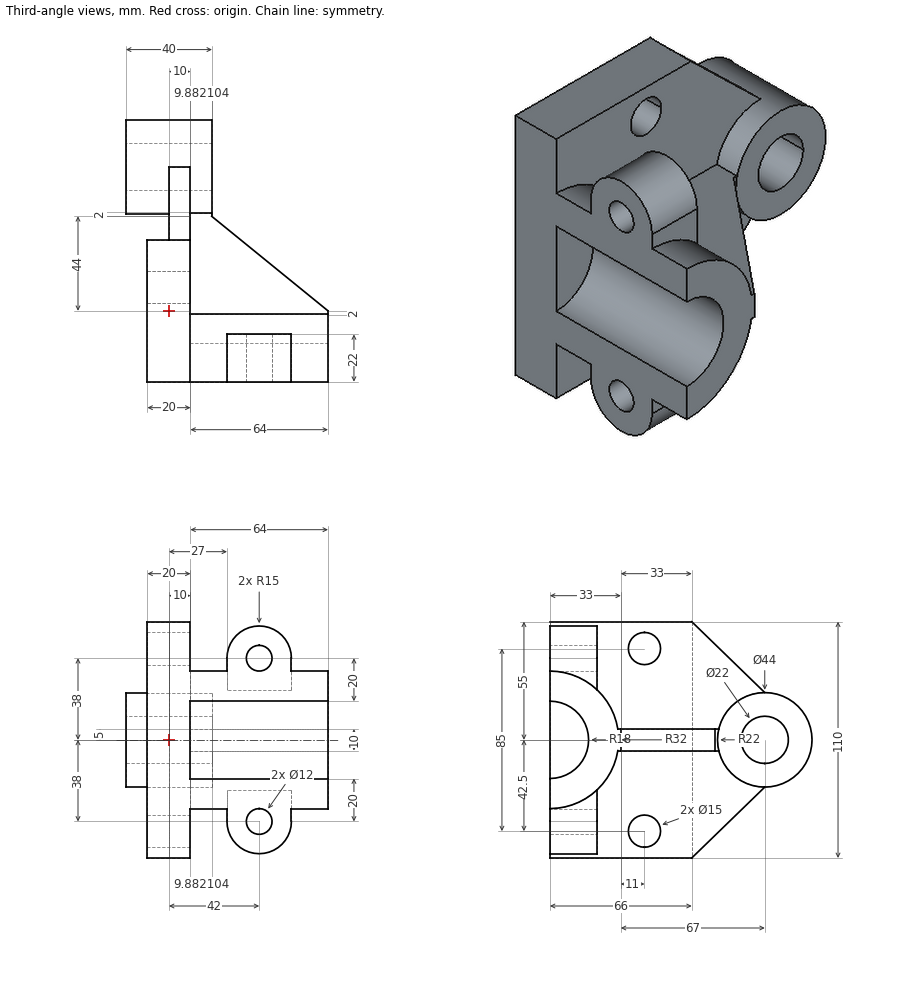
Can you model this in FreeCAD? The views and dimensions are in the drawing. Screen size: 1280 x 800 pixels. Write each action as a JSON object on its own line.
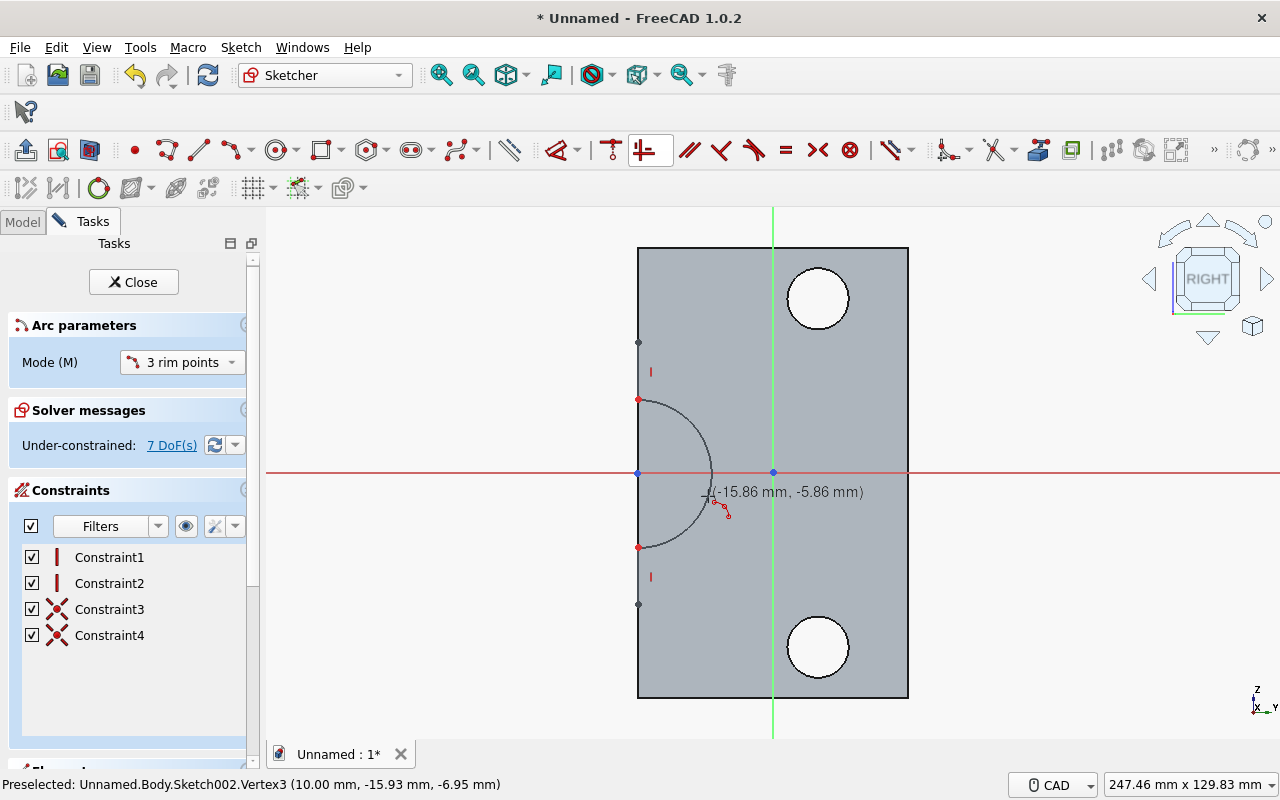
{"action": "left_click", "coordinate": [638, 605]}
{"action": "left_click", "coordinate": [638, 343]}
{"action": "left_click", "coordinate": [744, 550]}
{"action": "key", "text": "Escape"}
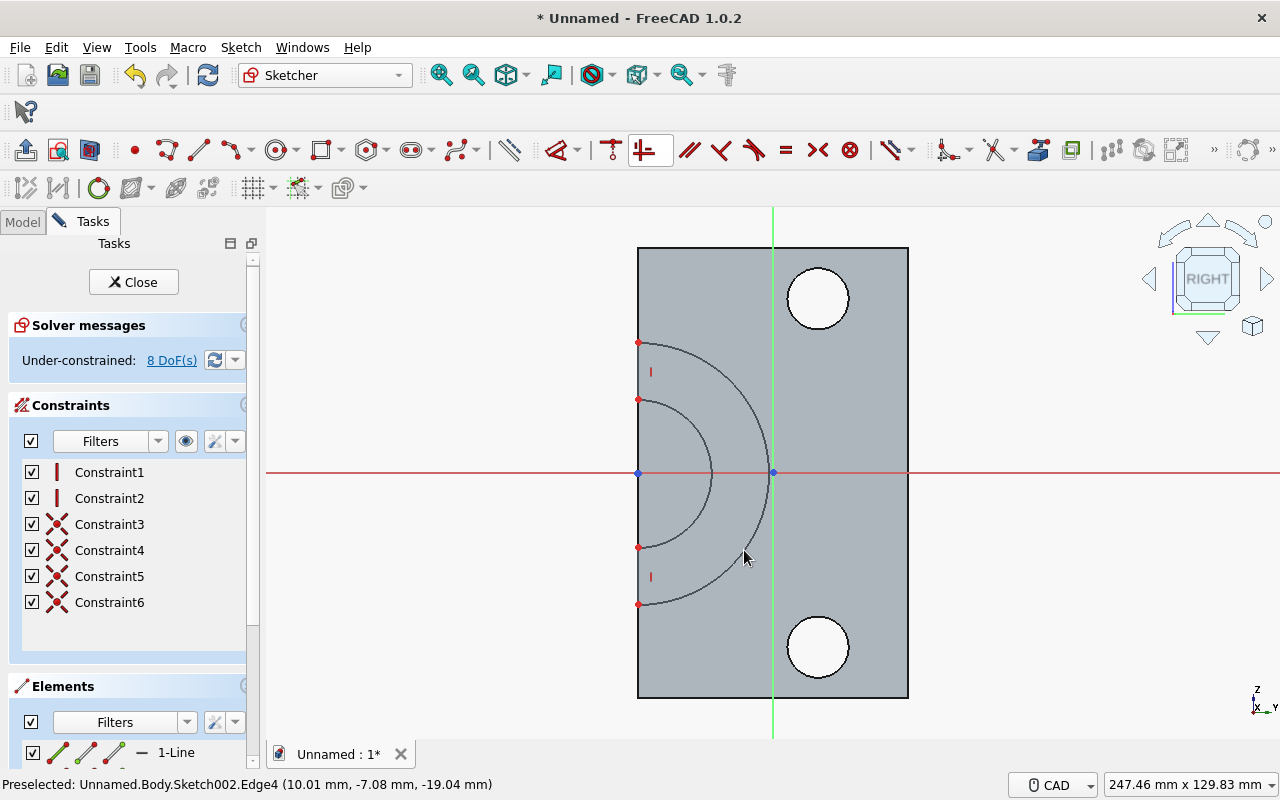
{"action": "left_click", "coordinate": [698, 517]}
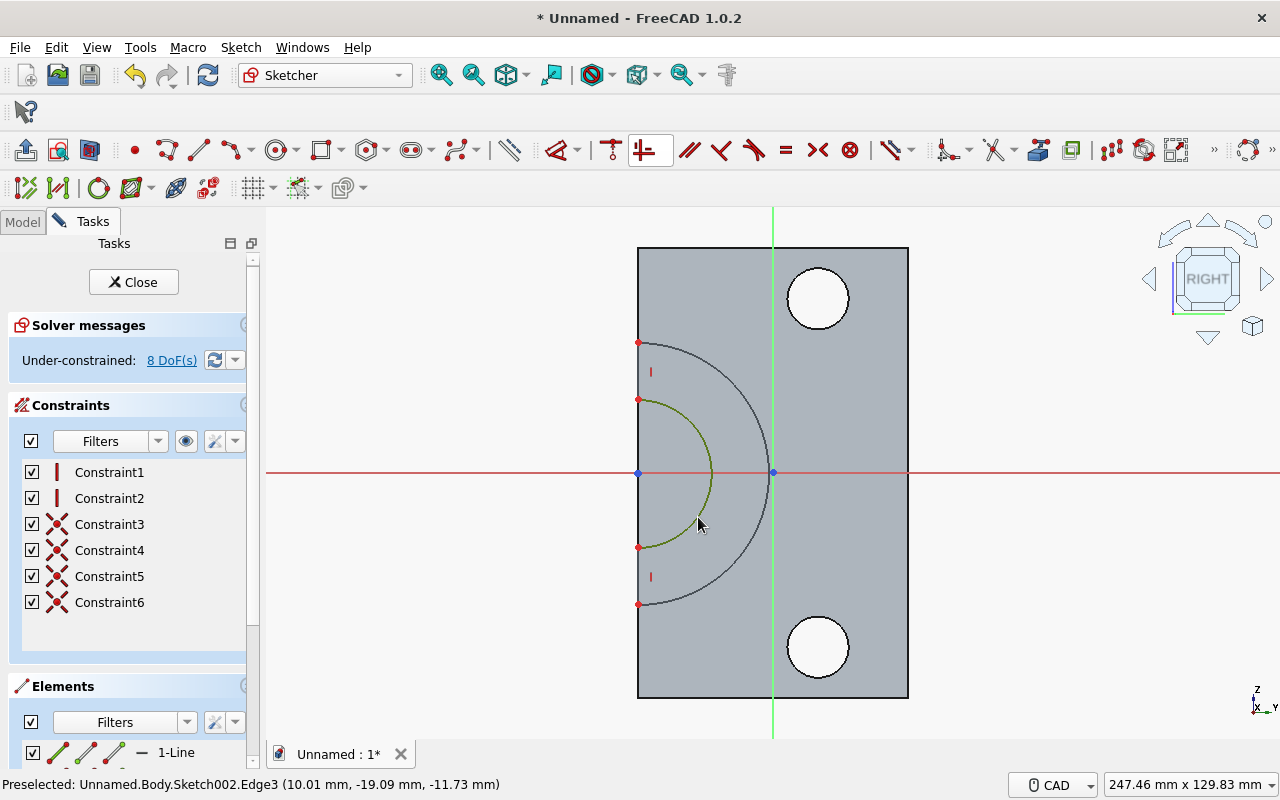
{"action": "left_click", "coordinate": [744, 551]}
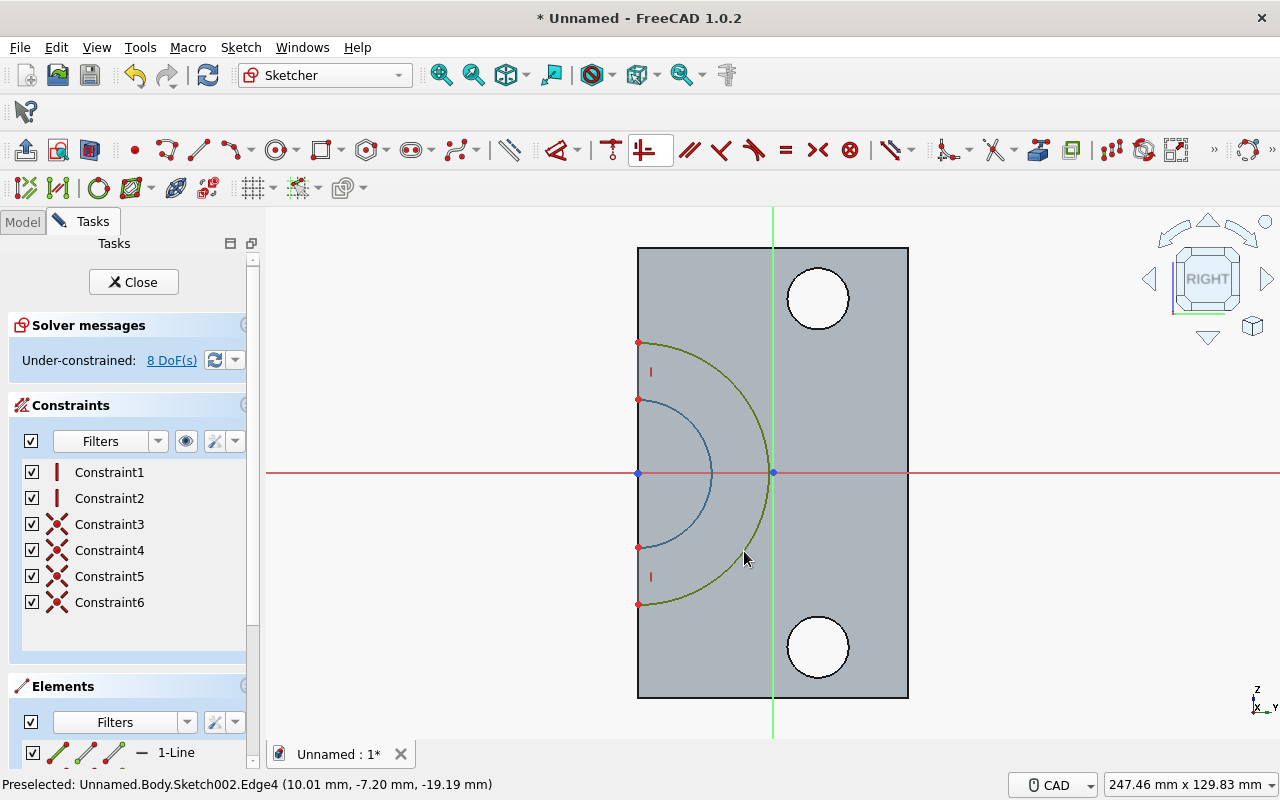
{"action": "left_click", "coordinate": [612, 150]}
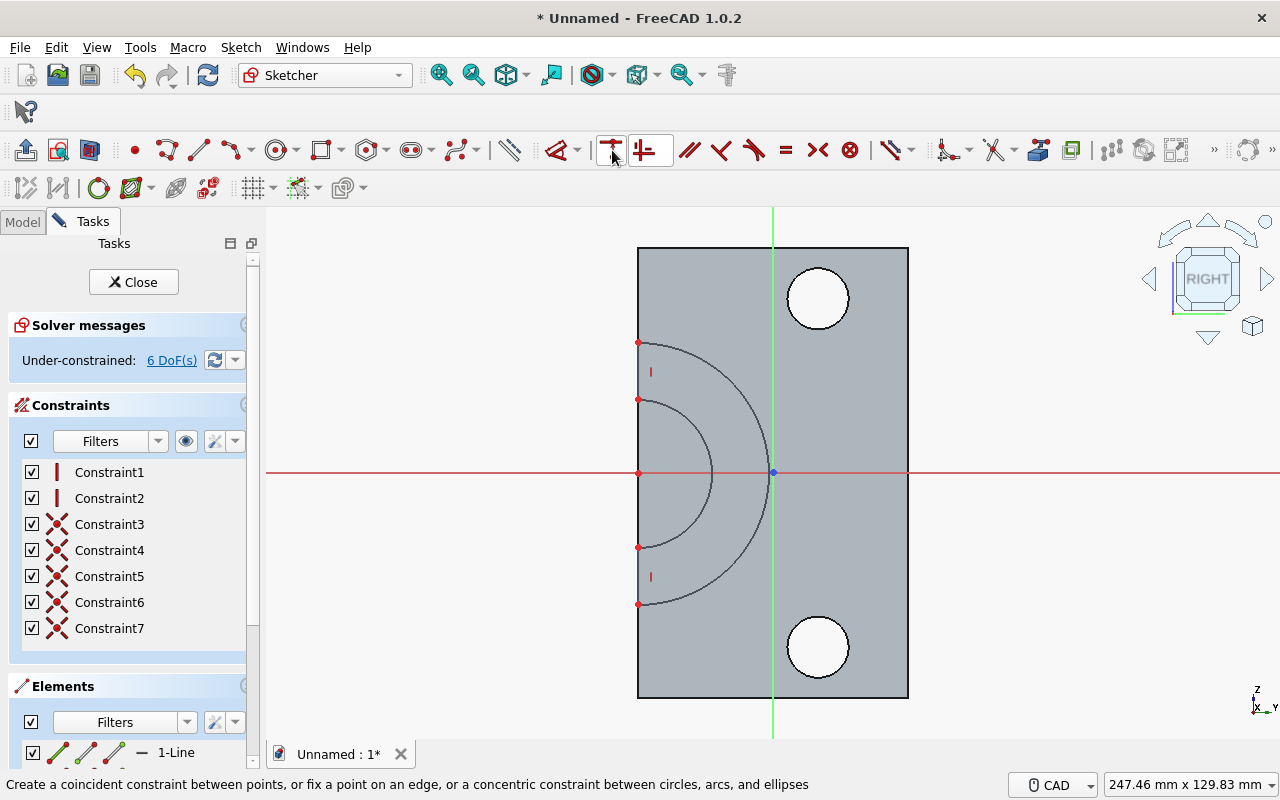
{"action": "left_click", "coordinate": [638, 474]}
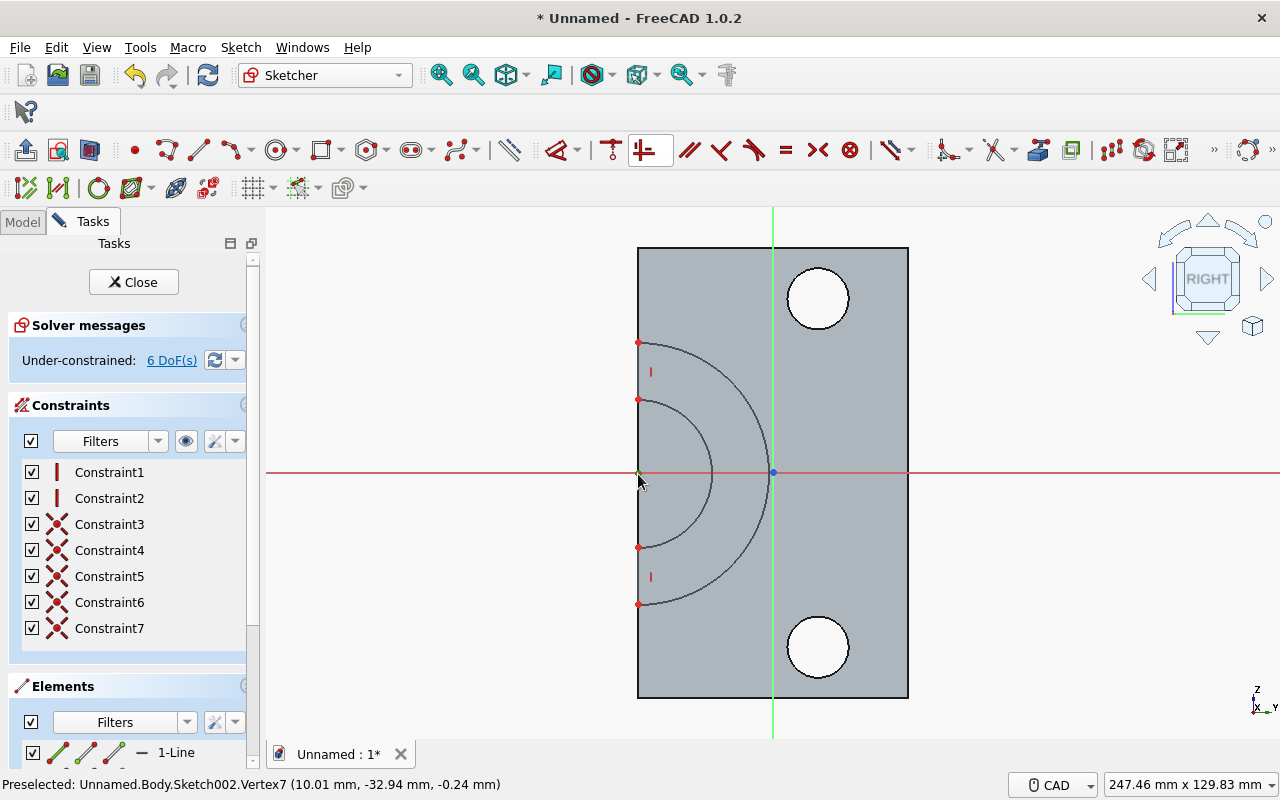
{"action": "left_click", "coordinate": [353, 473]}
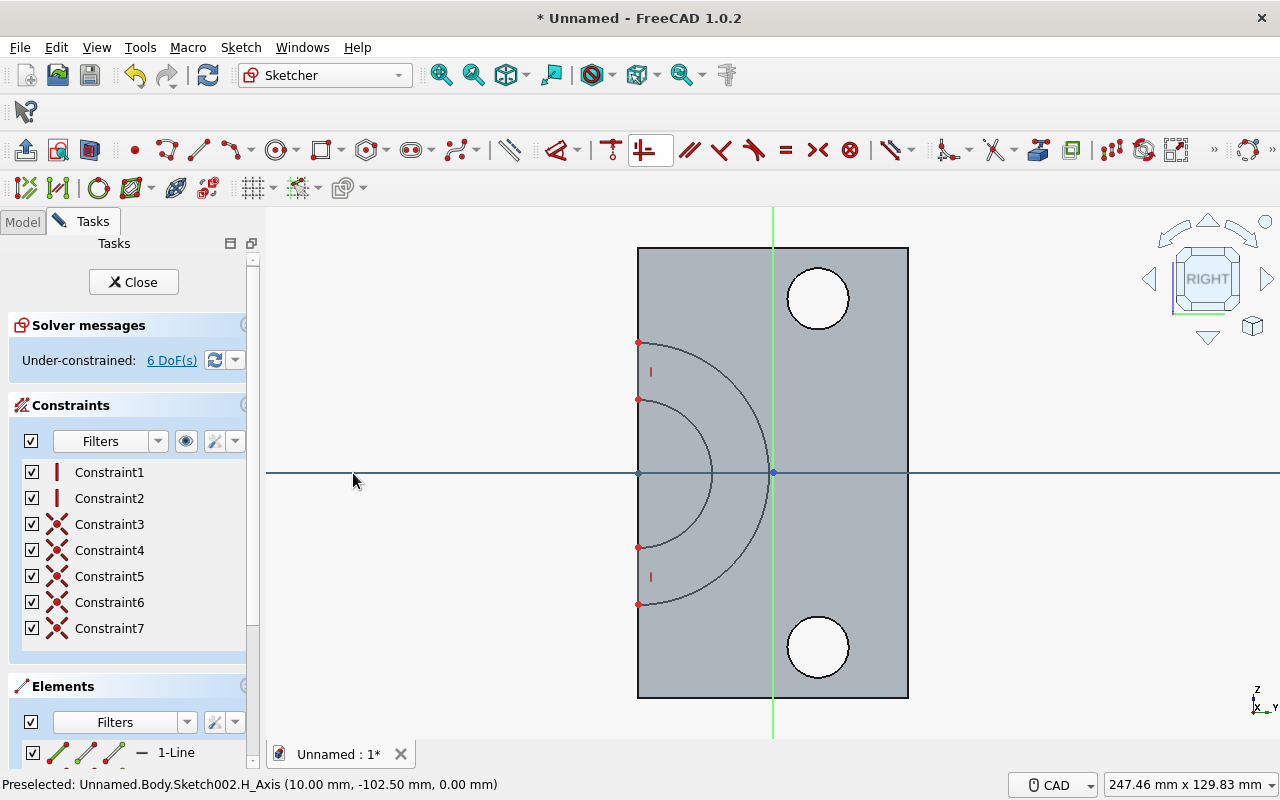
{"action": "key", "text": "c"}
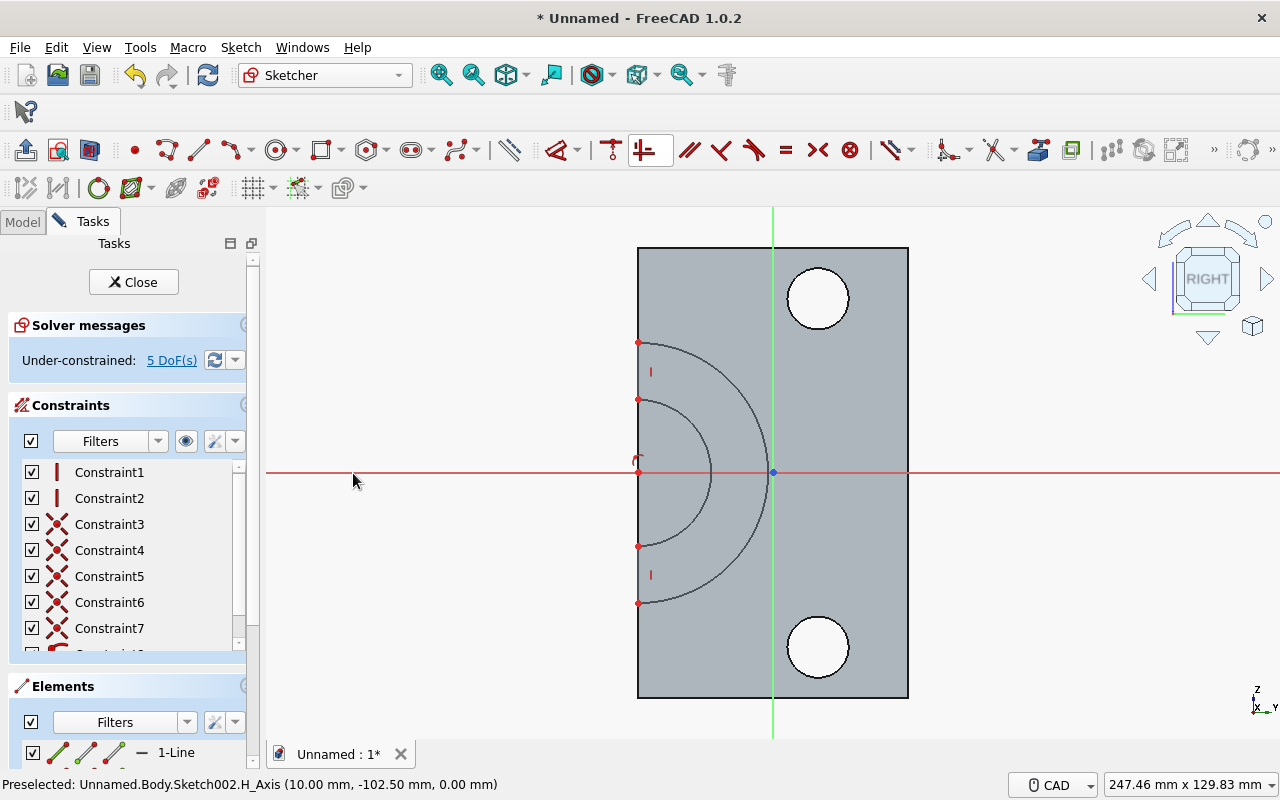
{"action": "left_click", "coordinate": [556, 150]}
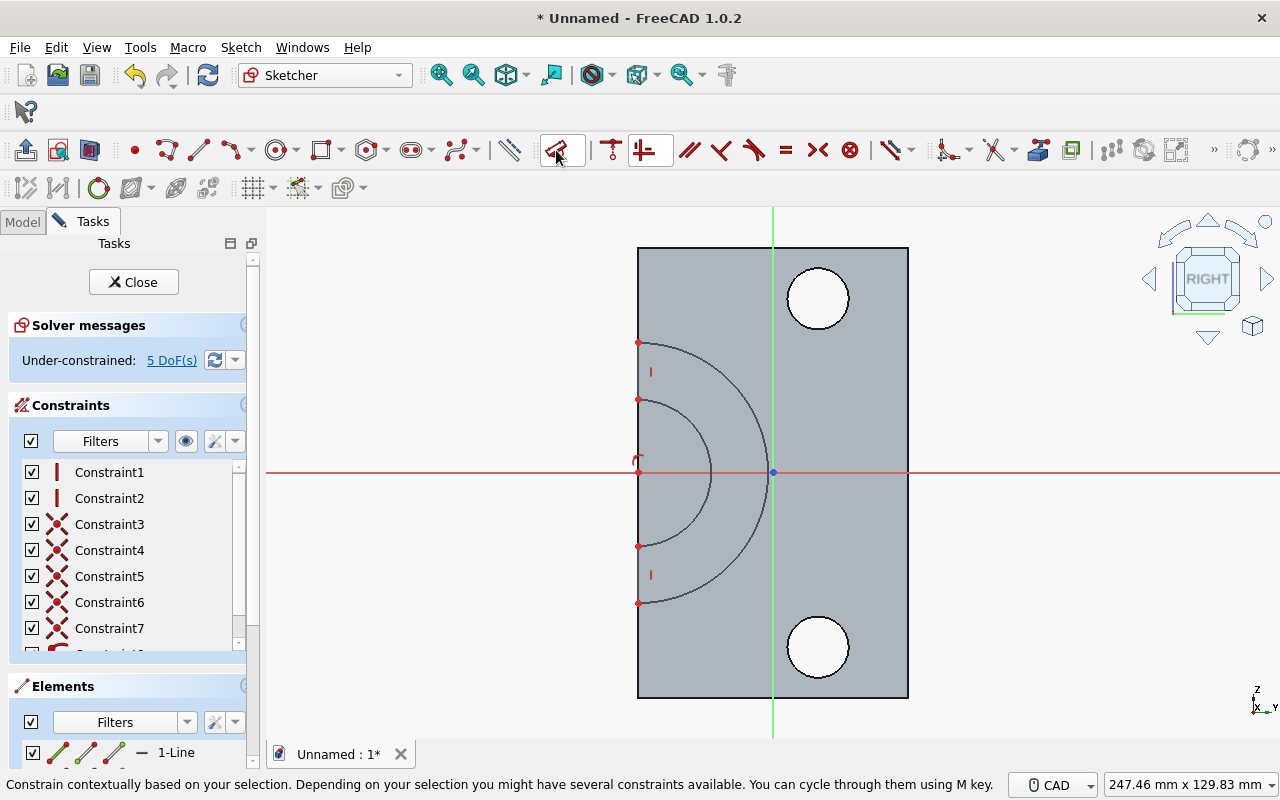
{"action": "left_click", "coordinate": [697, 516]}
{"action": "left_click", "coordinate": [723, 535]}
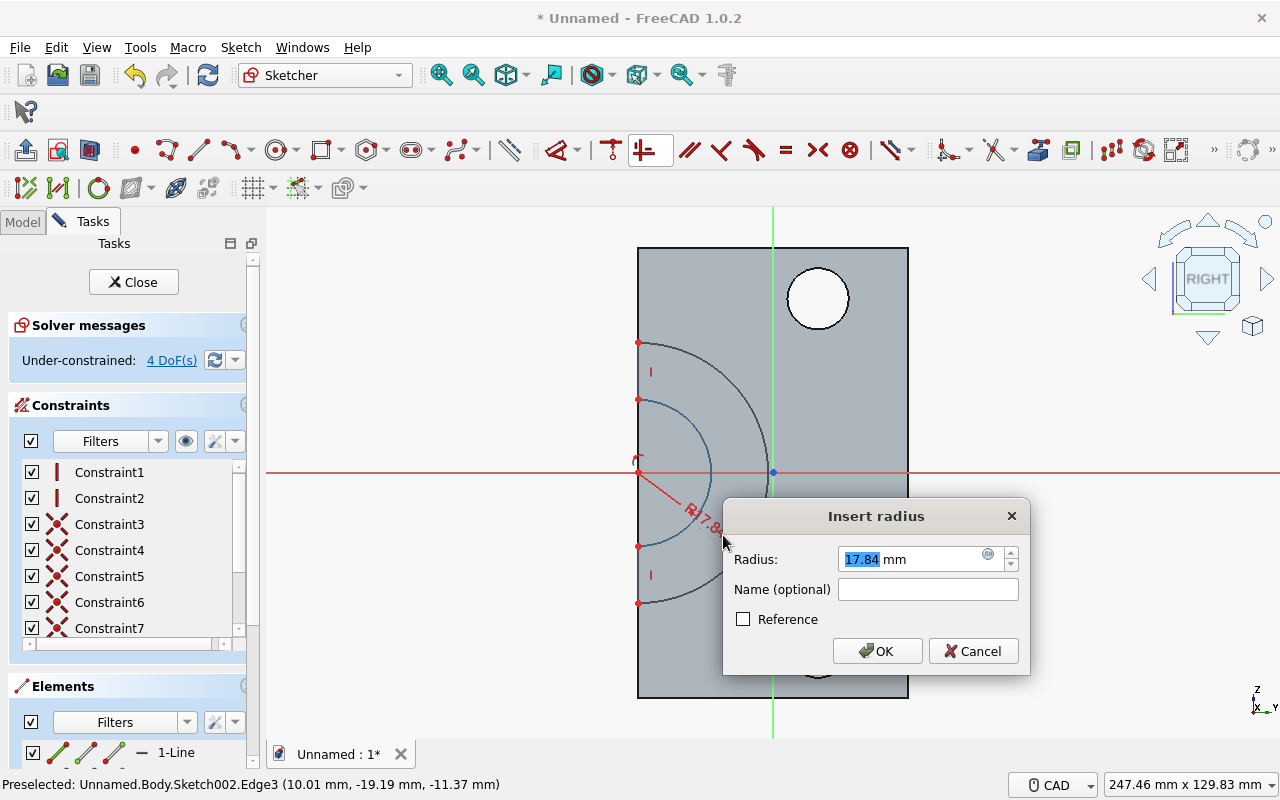
{"action": "type", "text": "18"}
{"action": "key", "text": "Return"}